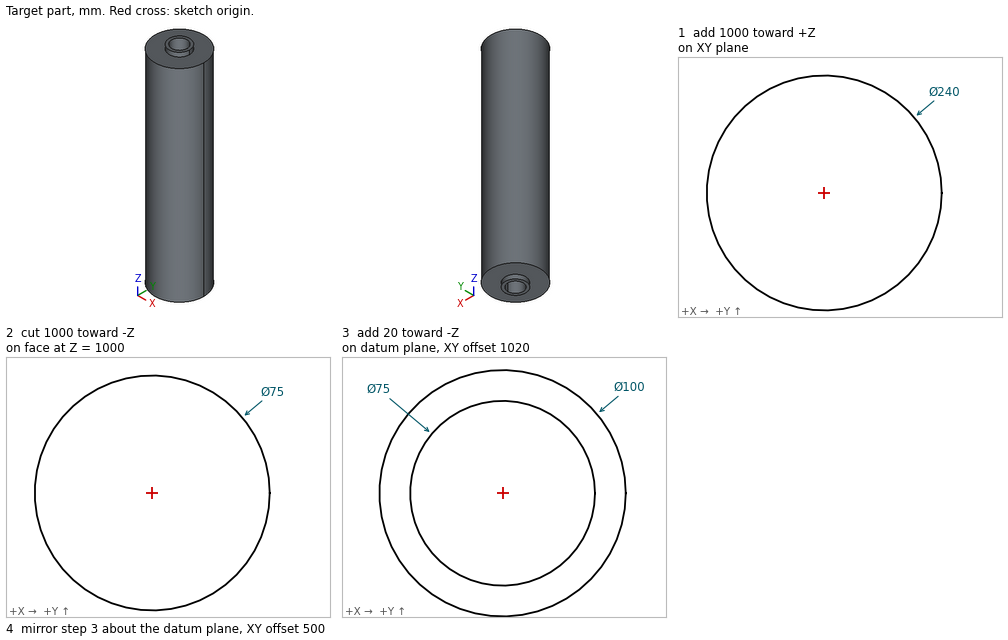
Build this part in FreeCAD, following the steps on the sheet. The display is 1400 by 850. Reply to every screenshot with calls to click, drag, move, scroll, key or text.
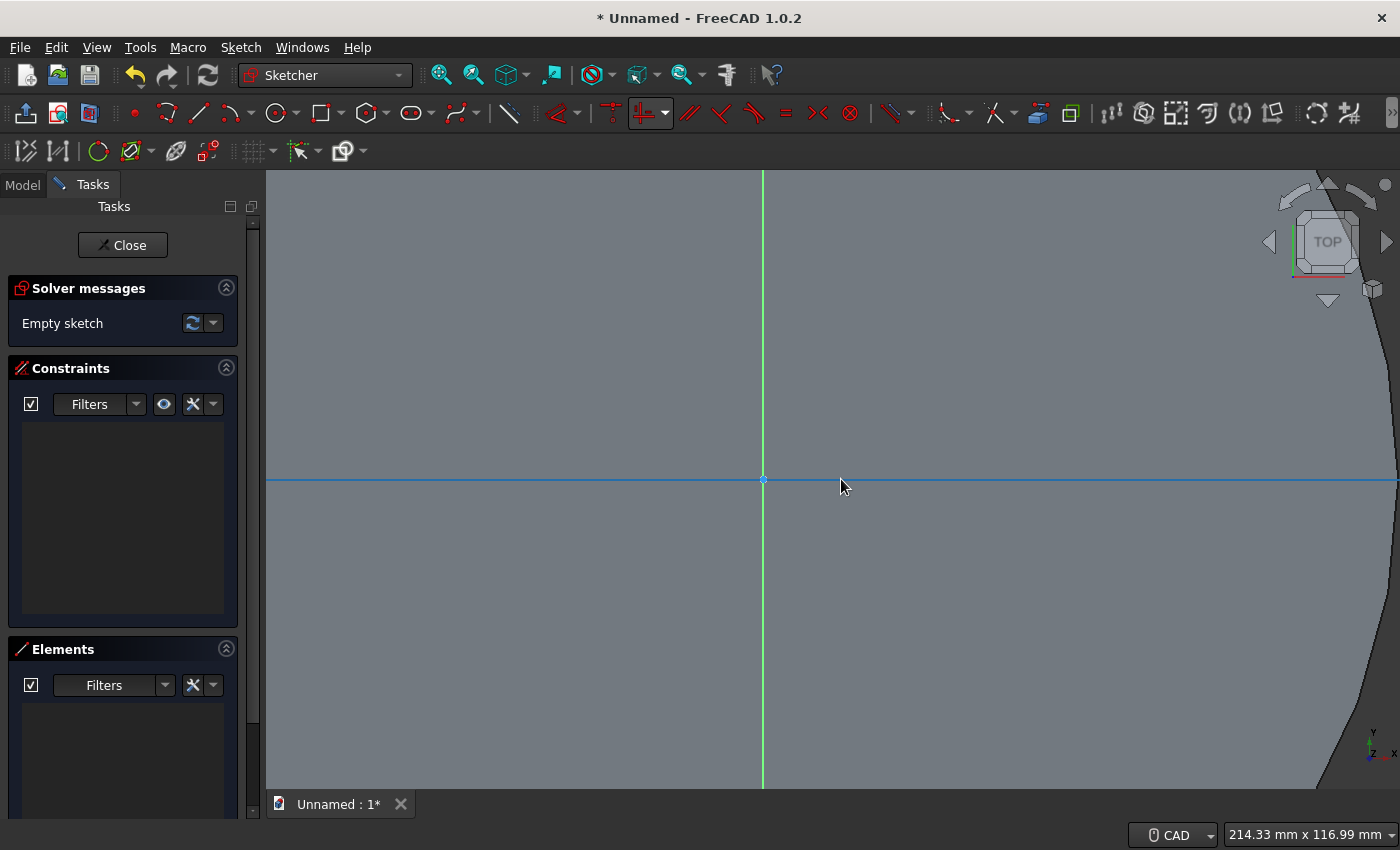
key(g)
key(c)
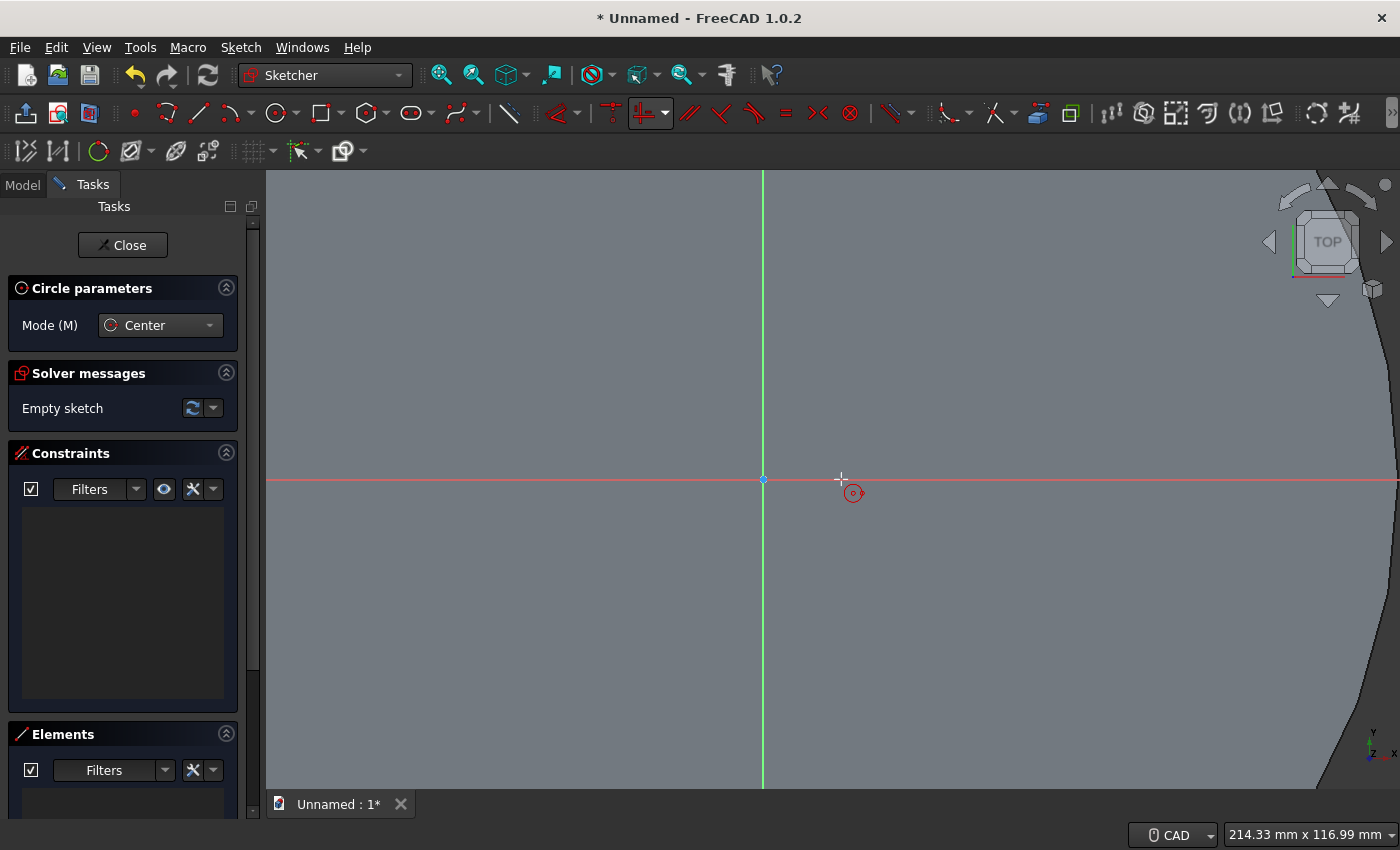
click(763, 480)
click(904, 339)
key(Escape)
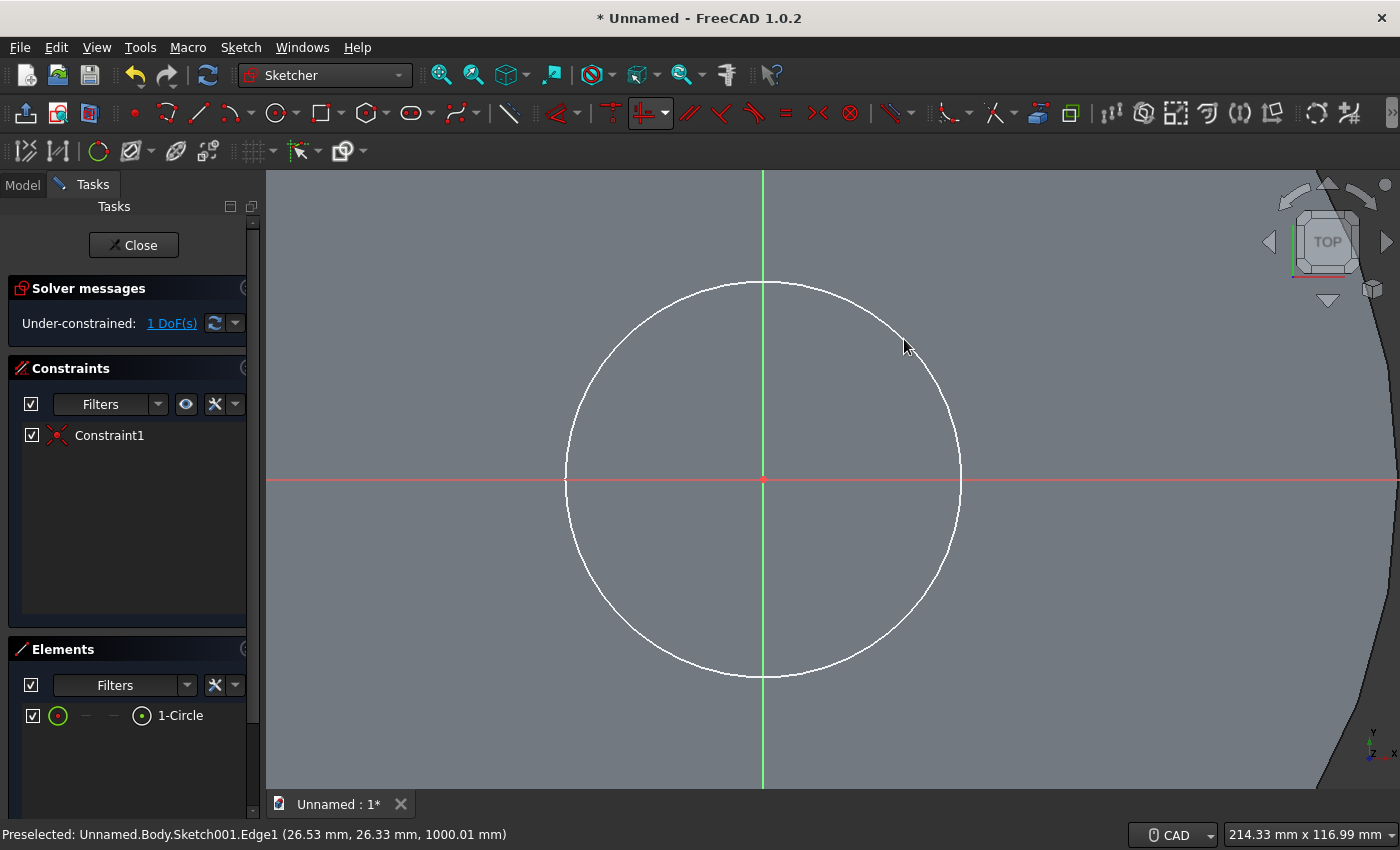
click(556, 114)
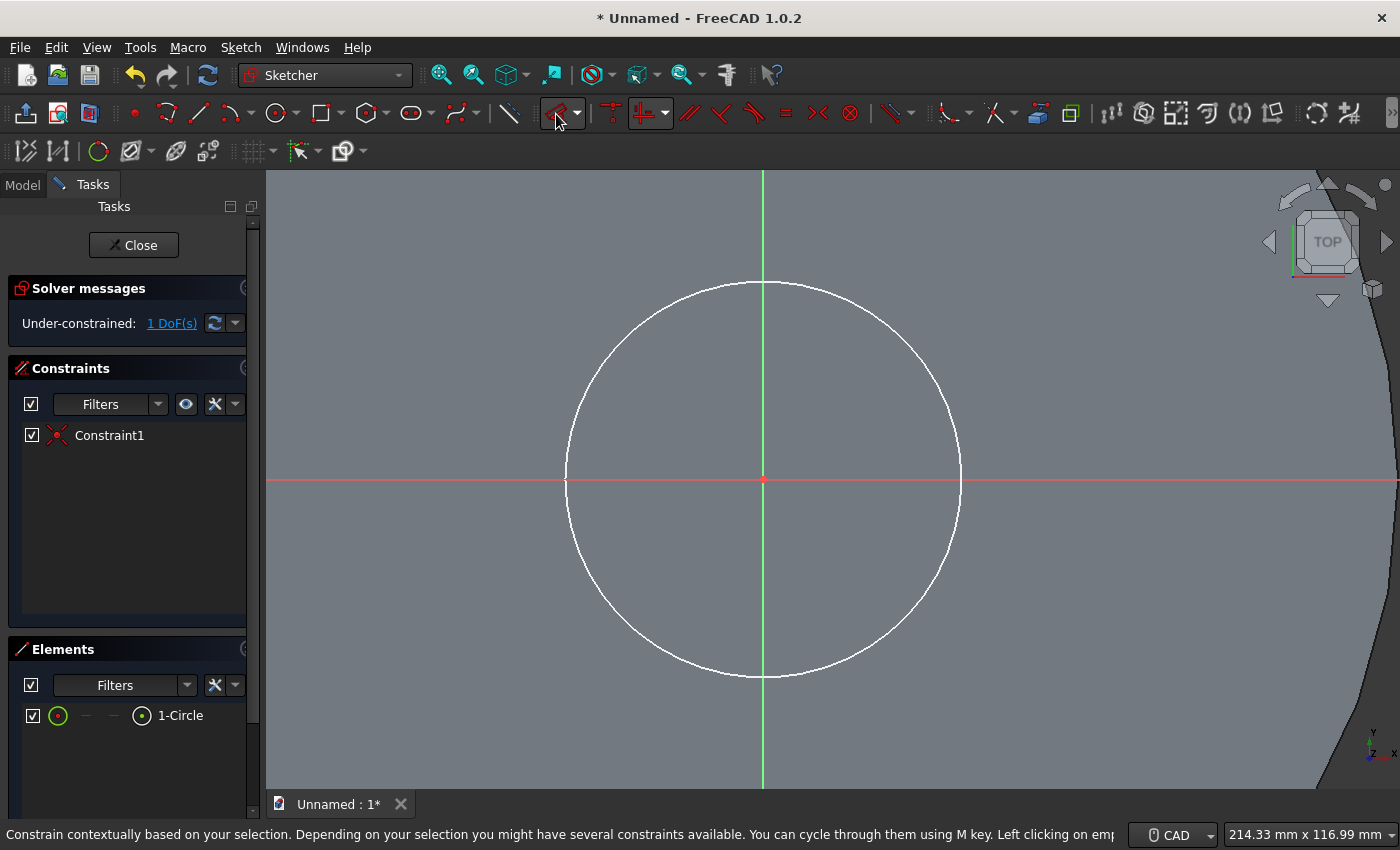
click(903, 339)
click(926, 316)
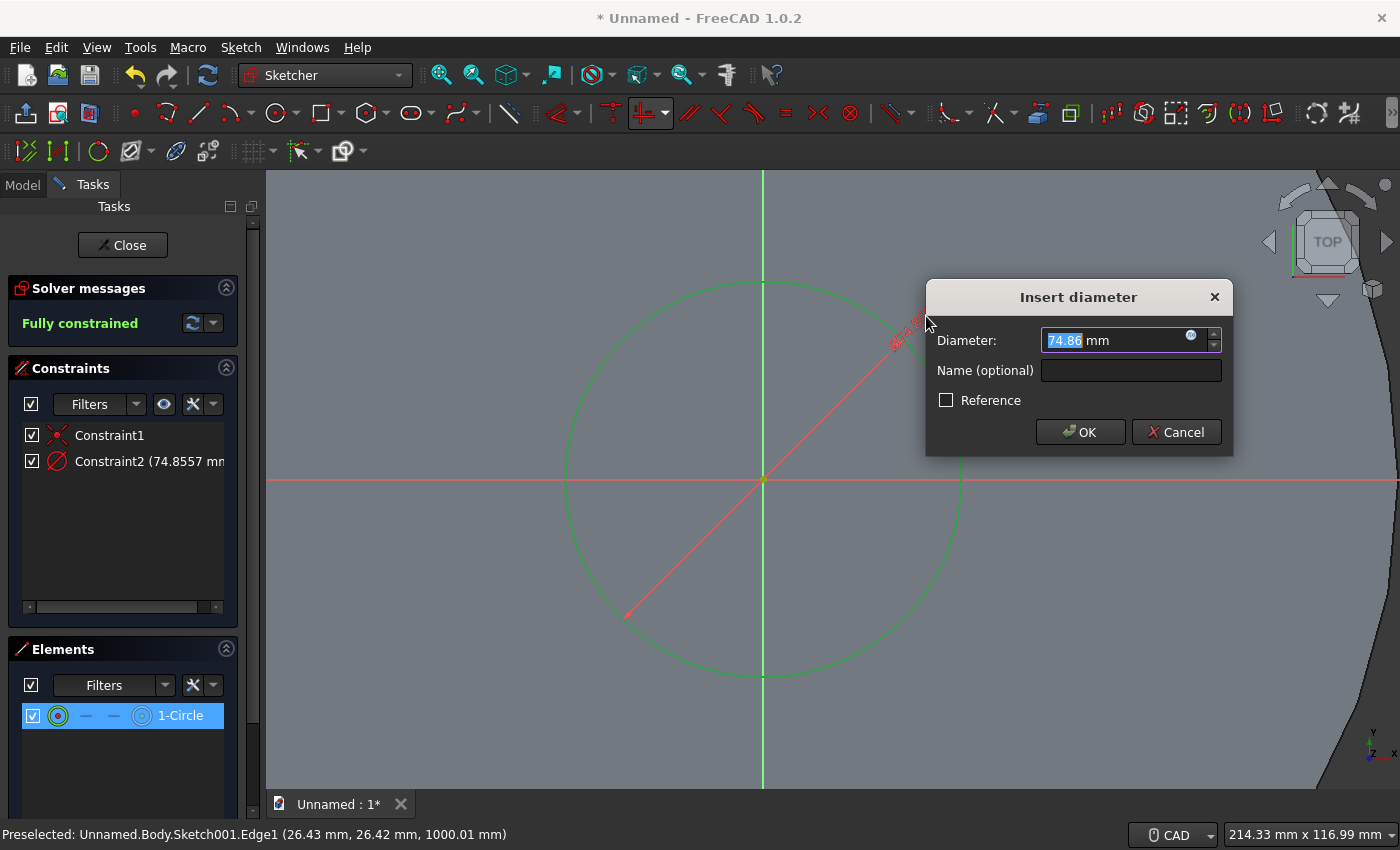
text(75)
key(Return)
key(Escape)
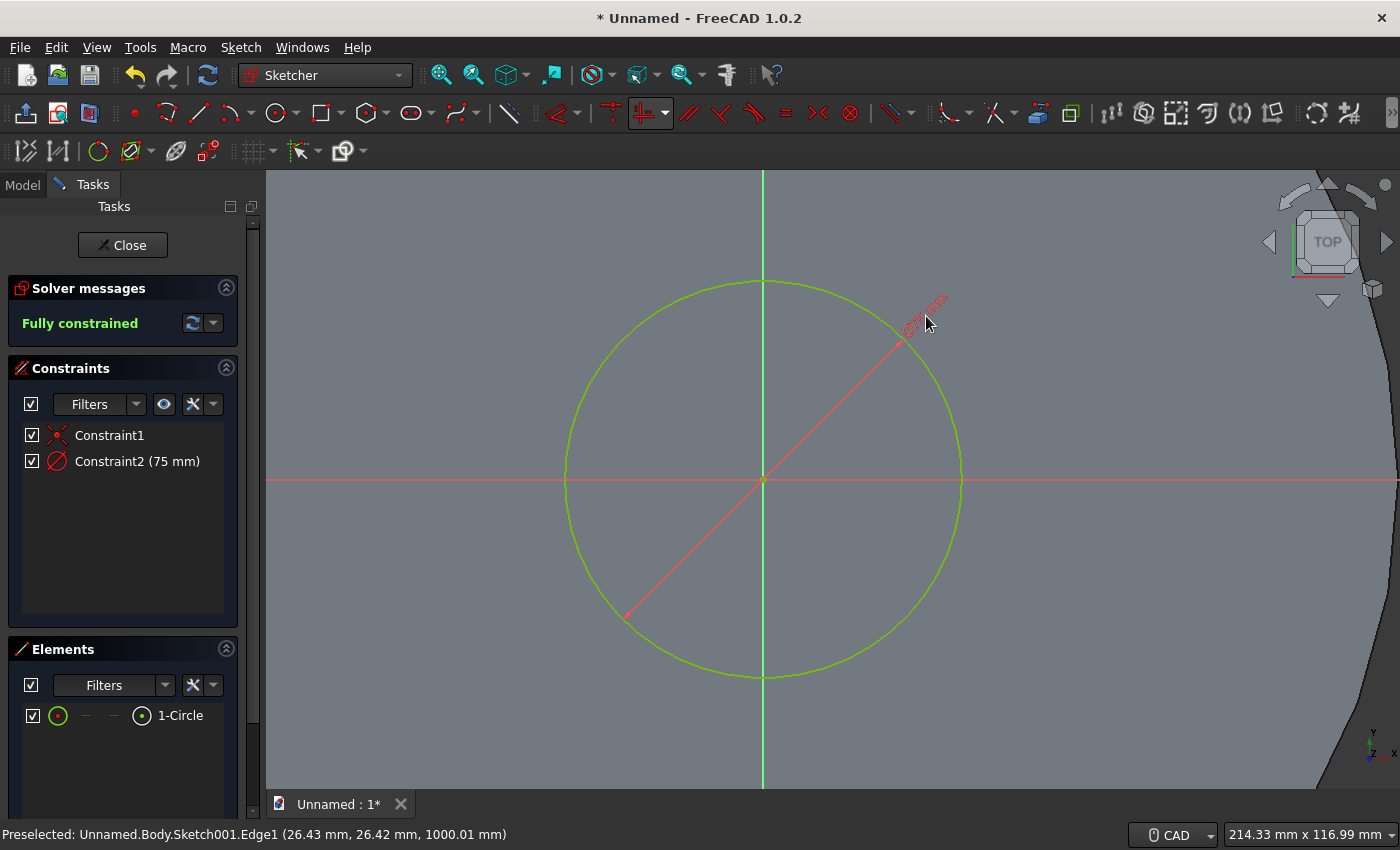
click(123, 245)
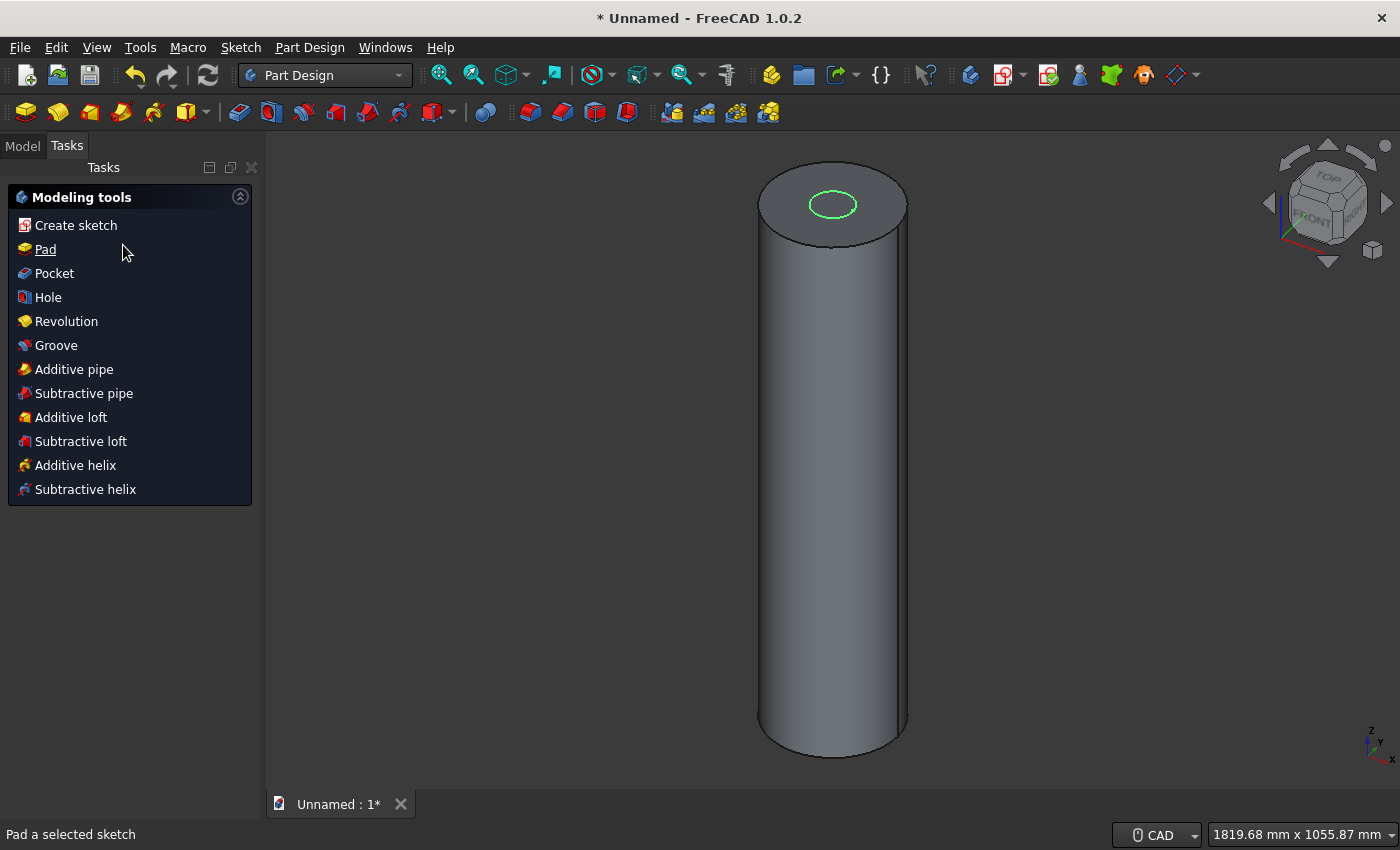
click(240, 112)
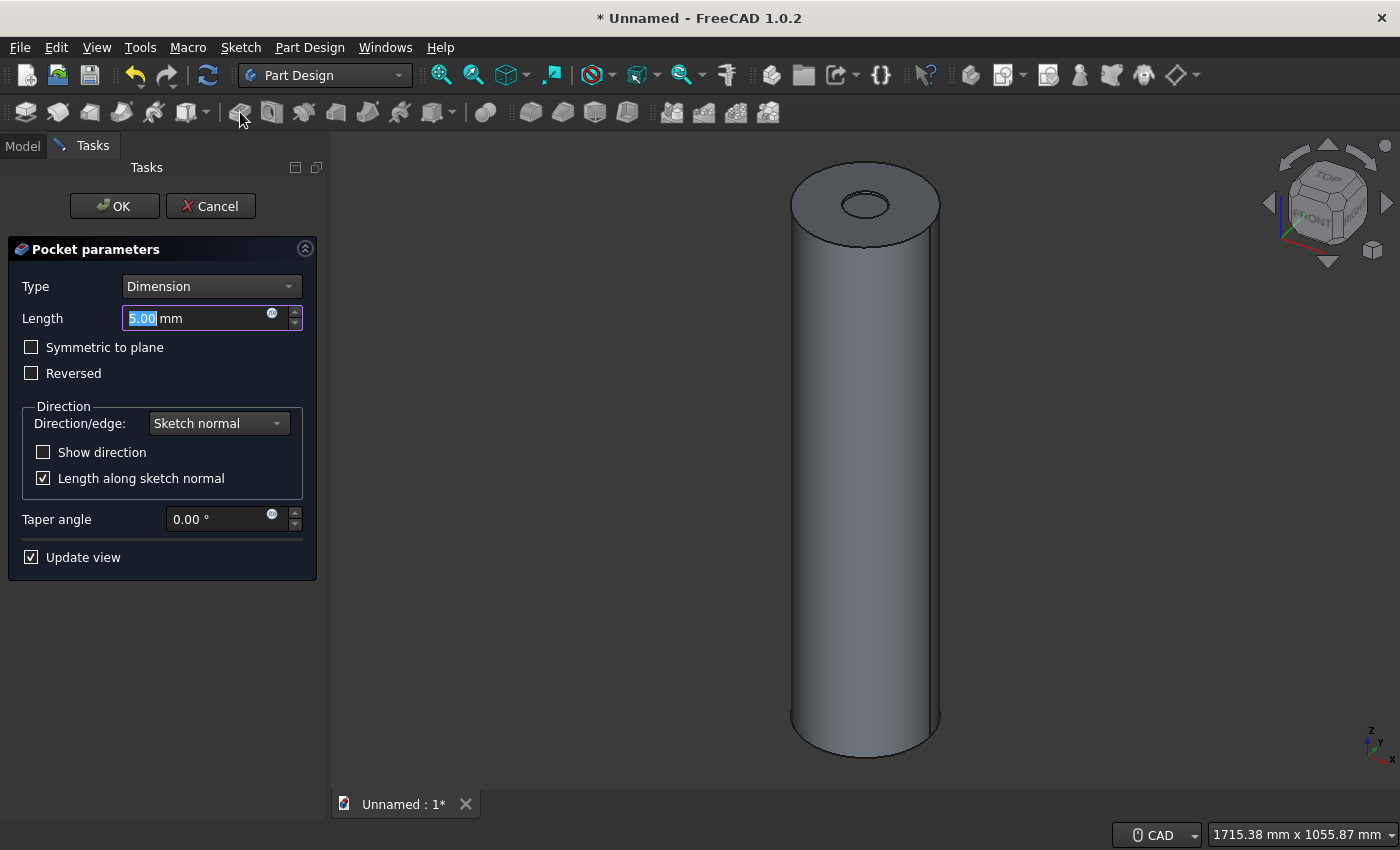
text(1000)
key(Tab)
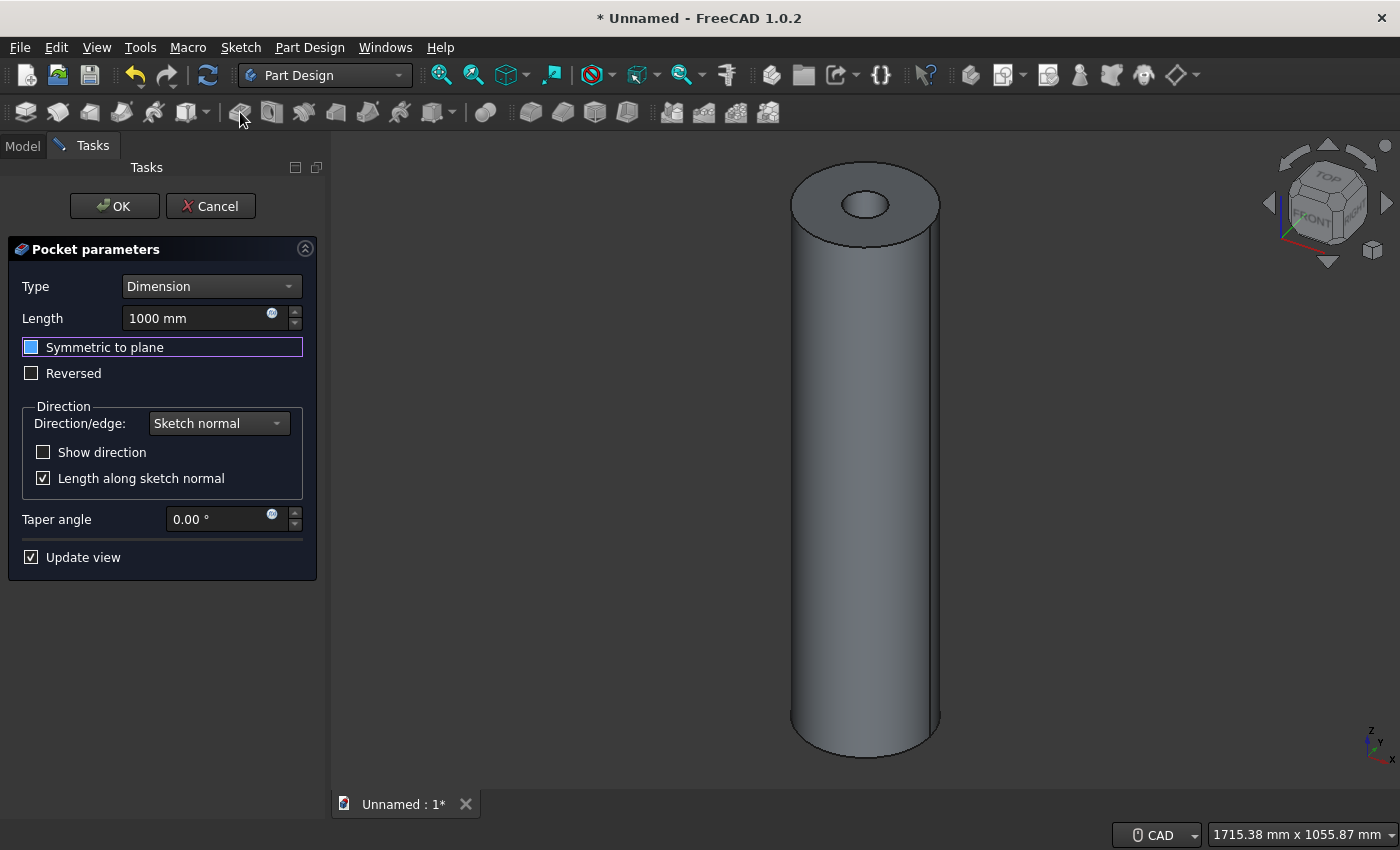
click(115, 206)